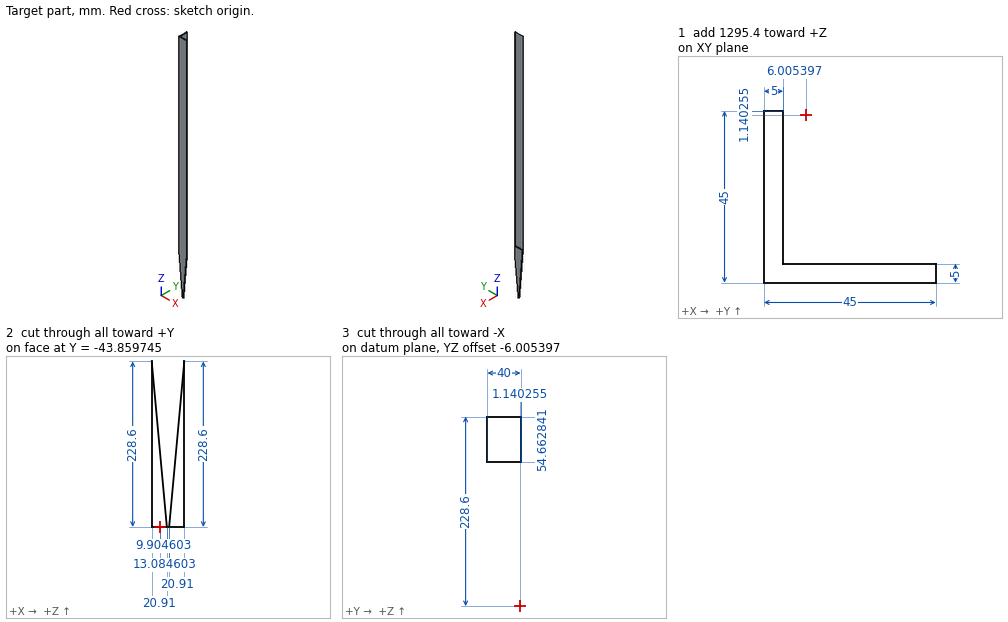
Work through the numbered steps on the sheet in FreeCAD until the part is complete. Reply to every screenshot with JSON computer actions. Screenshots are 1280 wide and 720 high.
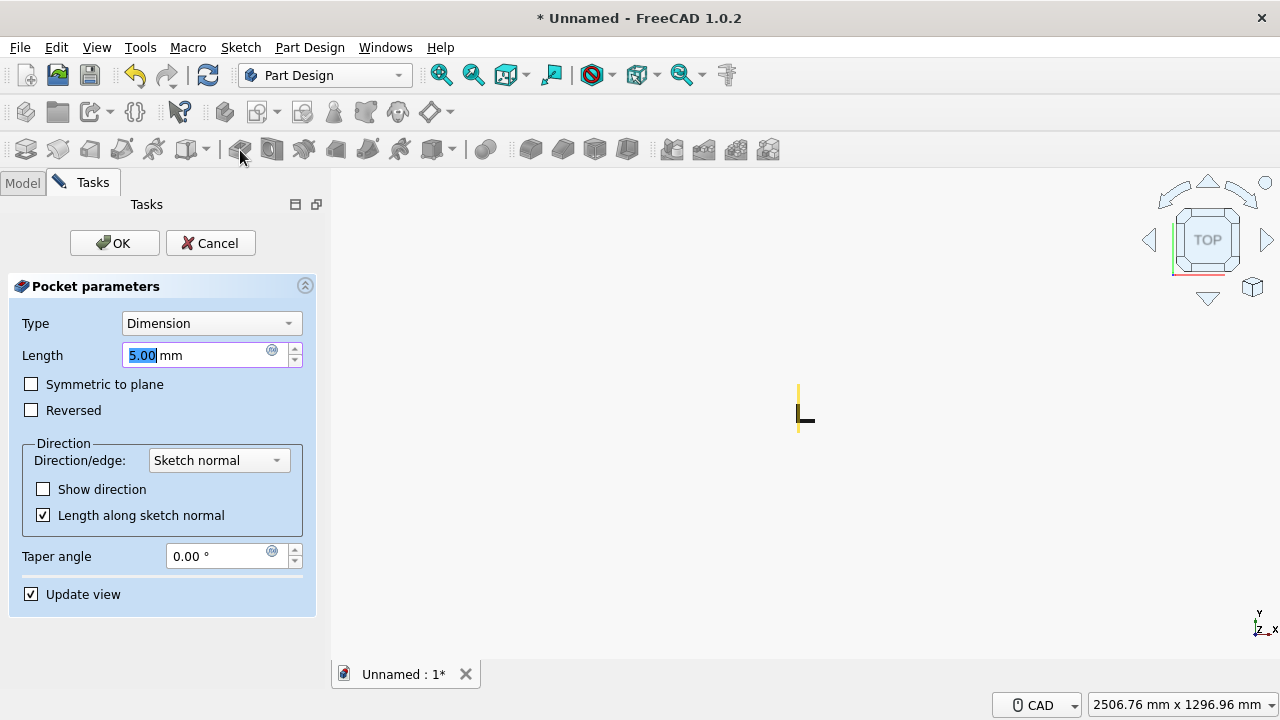
{"action": "left_click", "coordinate": [212, 324]}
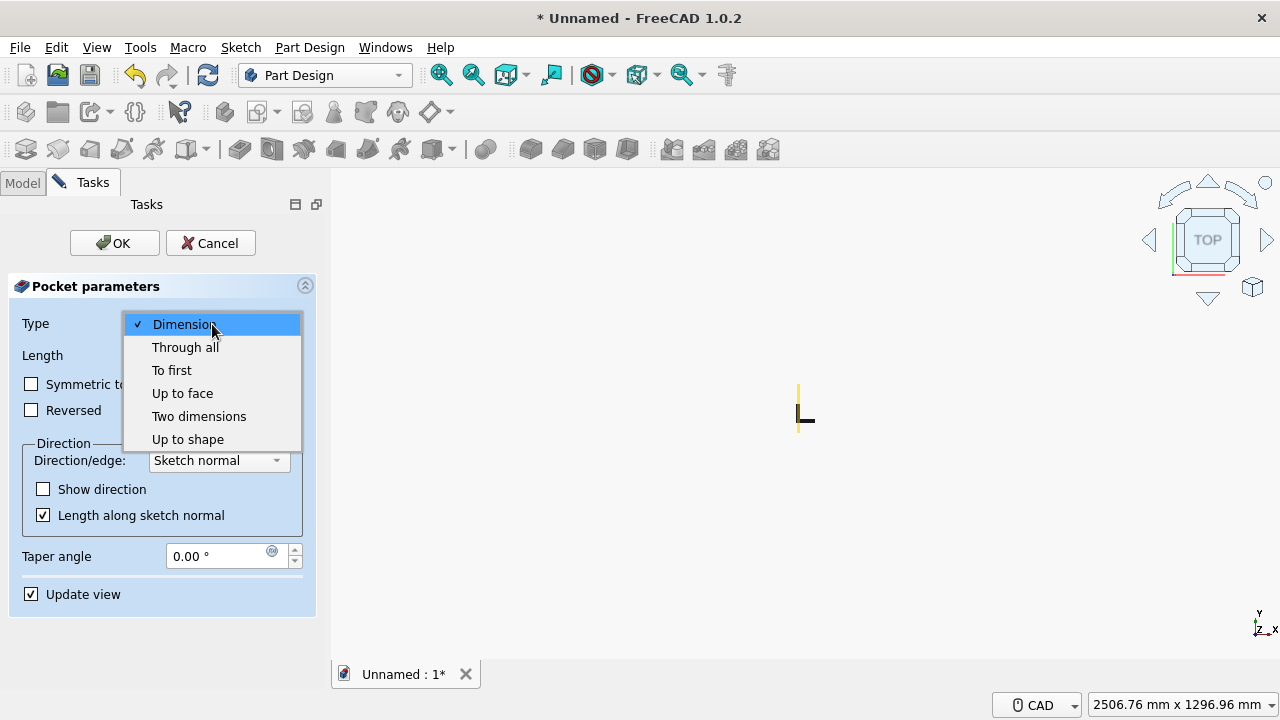
{"action": "left_click", "coordinate": [212, 348]}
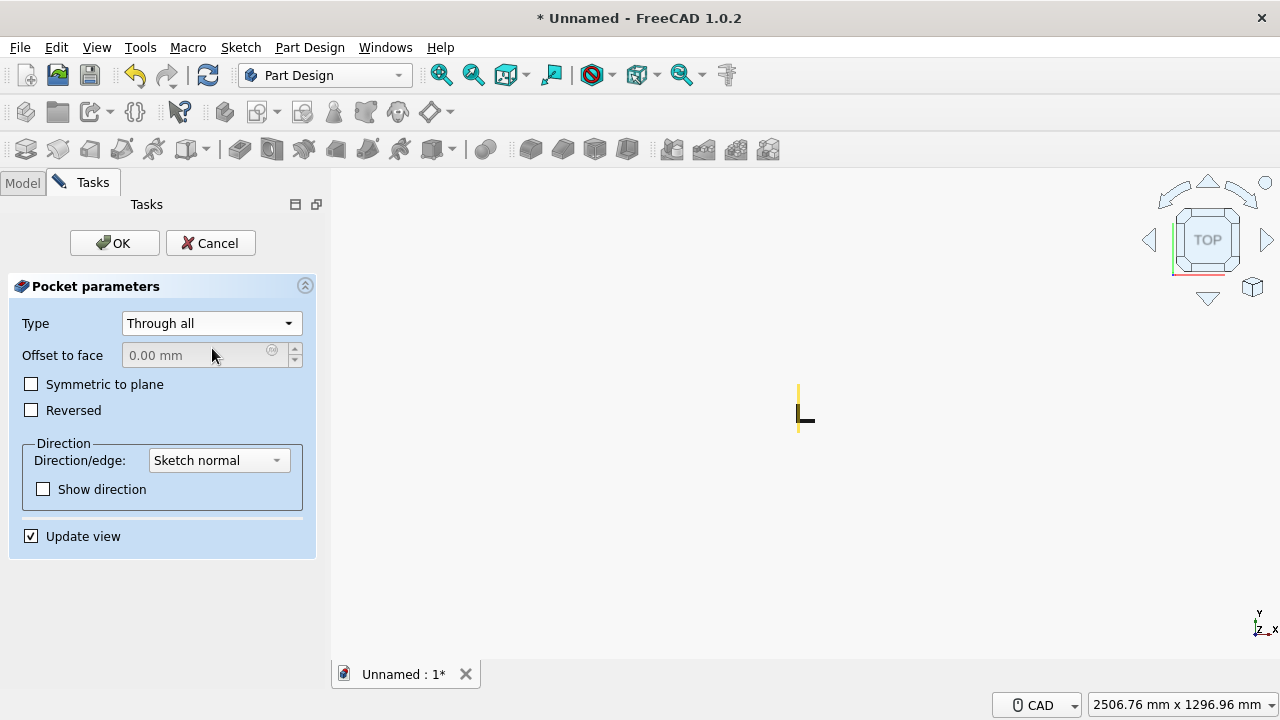
{"action": "left_click", "coordinate": [115, 243]}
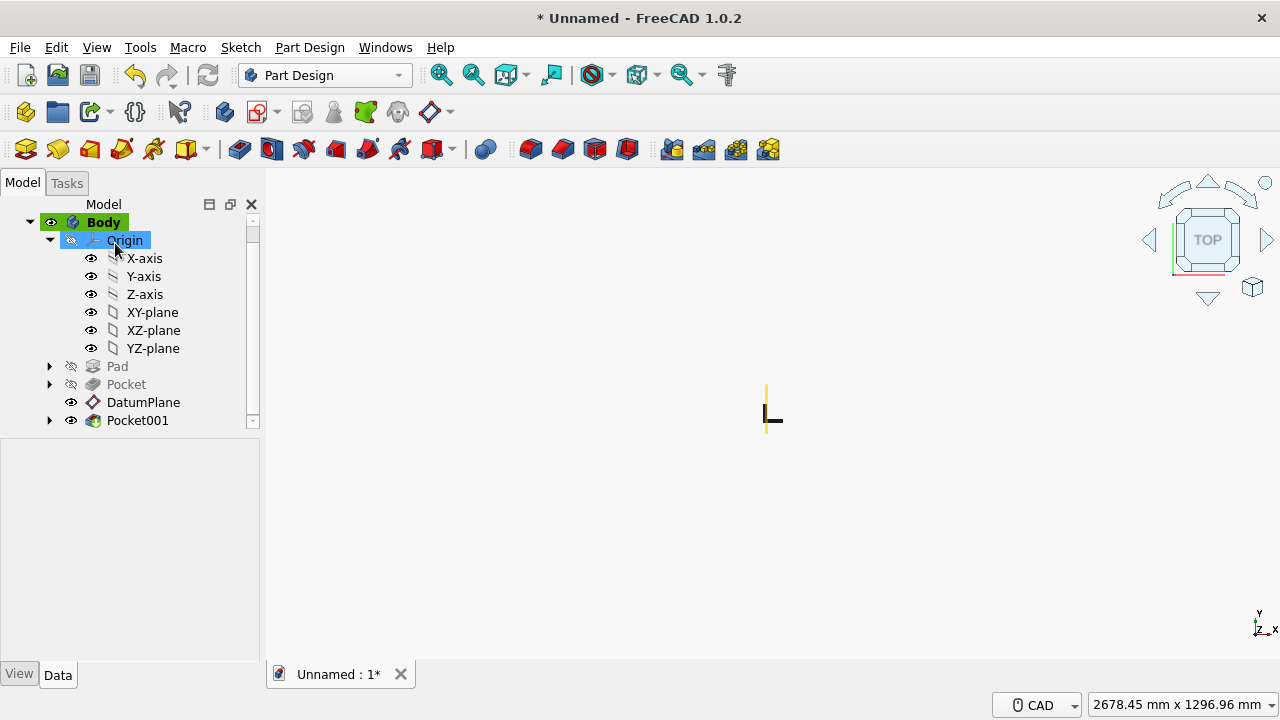
{"action": "left_click", "coordinate": [116, 402]}
{"action": "key", "text": "space"}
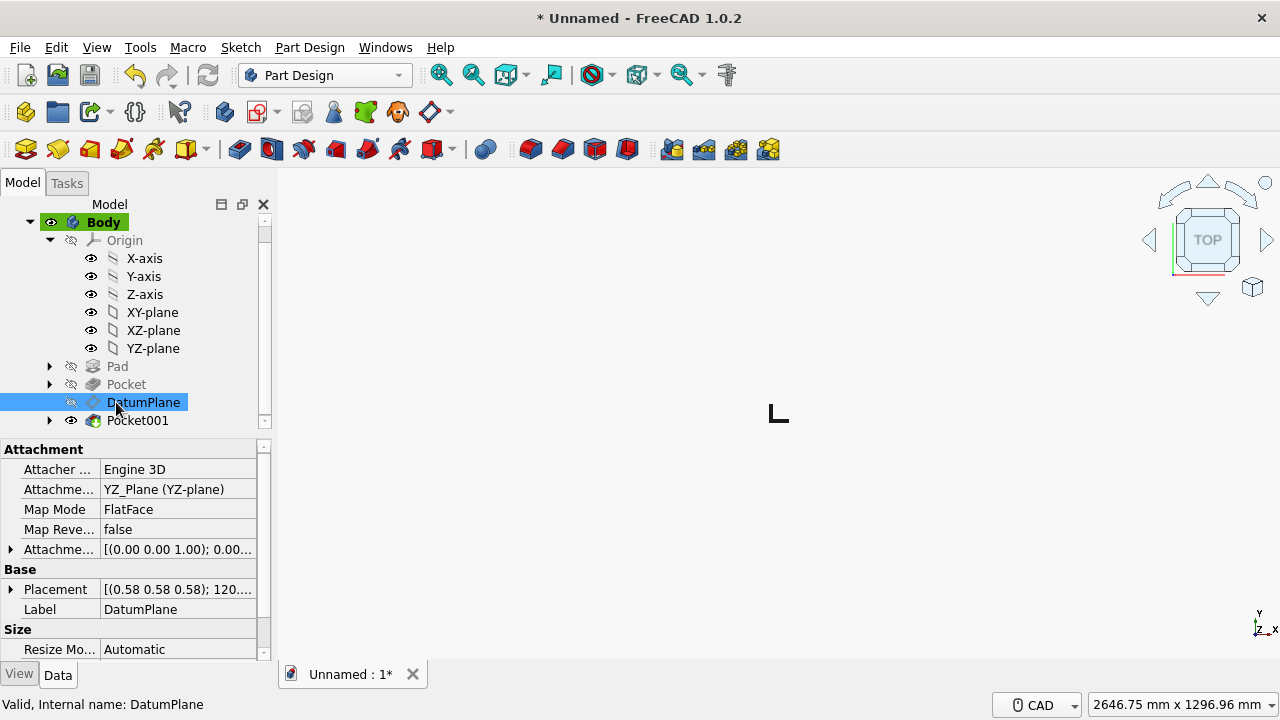
{"action": "key", "text": "0"}